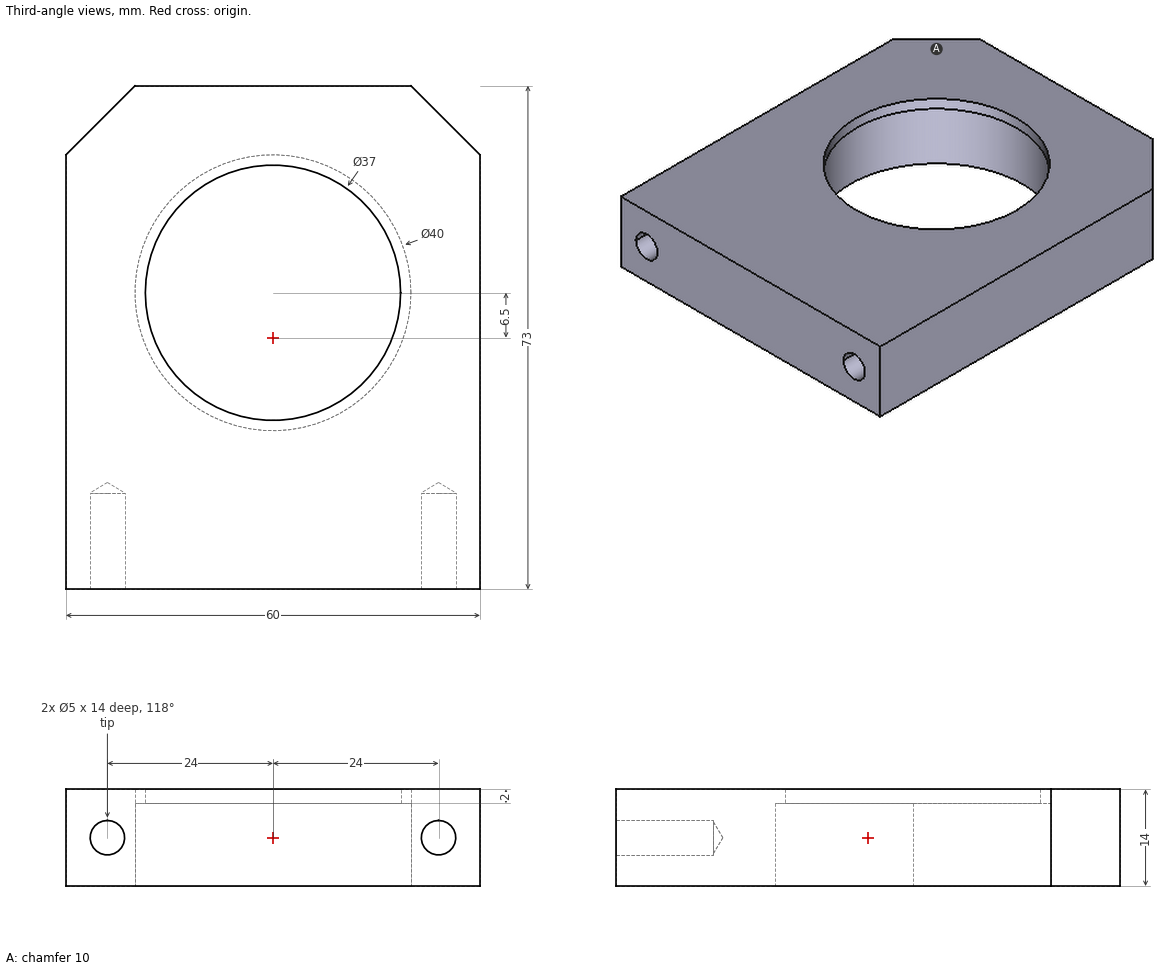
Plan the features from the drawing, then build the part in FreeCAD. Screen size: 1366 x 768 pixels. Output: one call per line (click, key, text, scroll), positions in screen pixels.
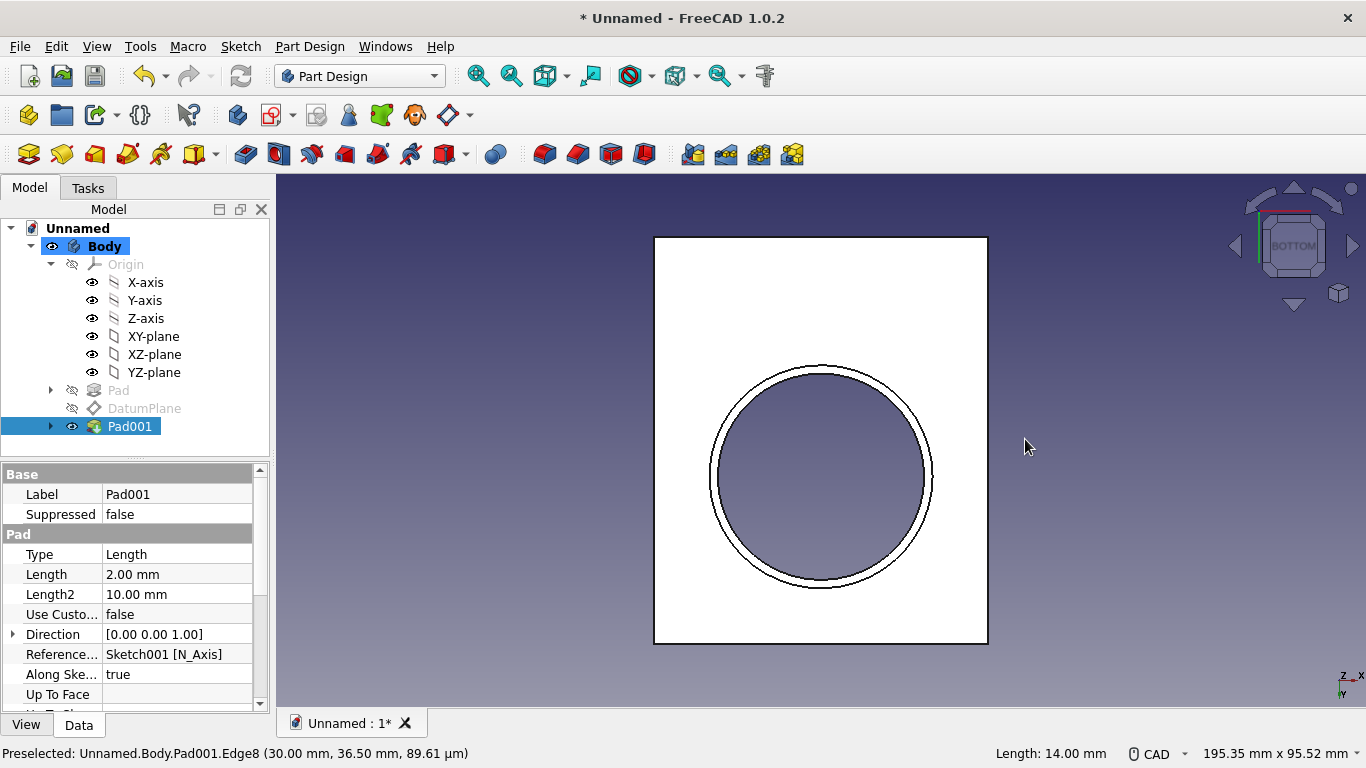
key(4)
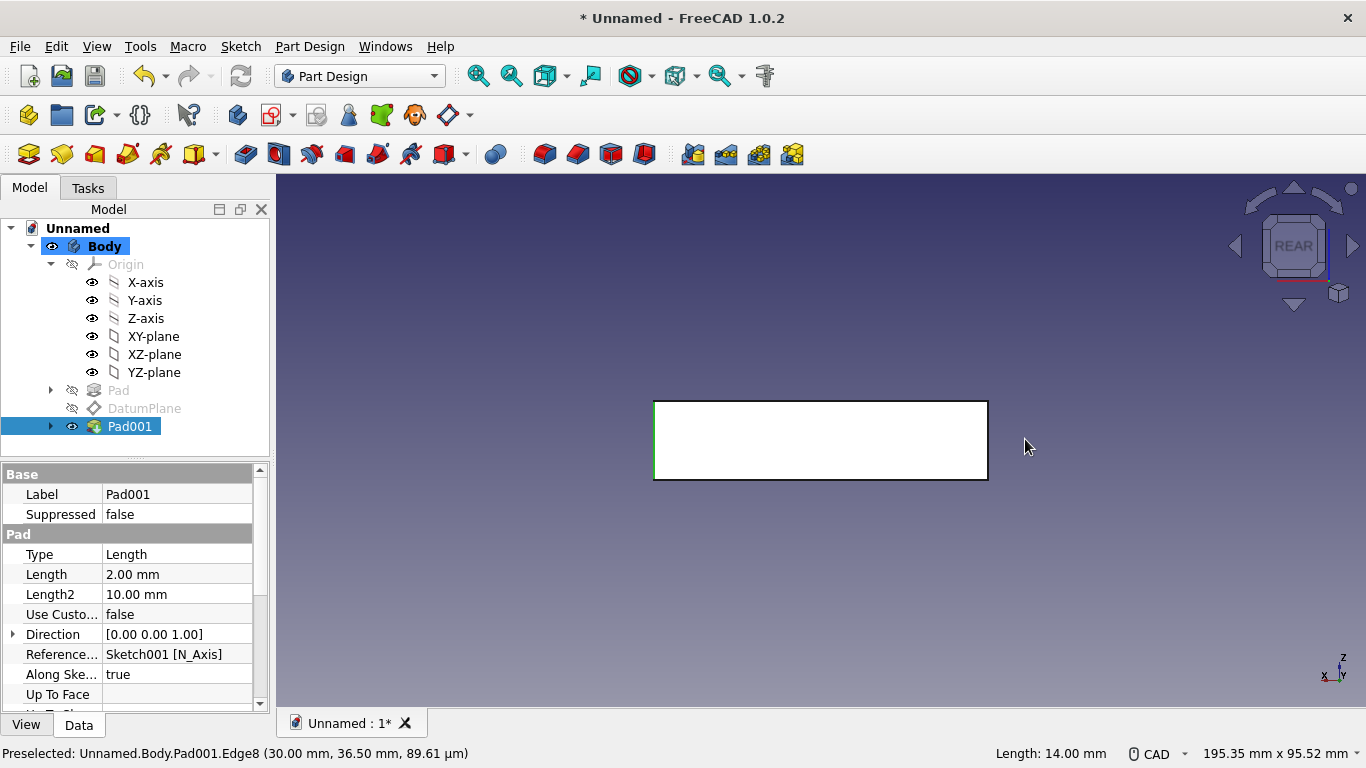
click(479, 76)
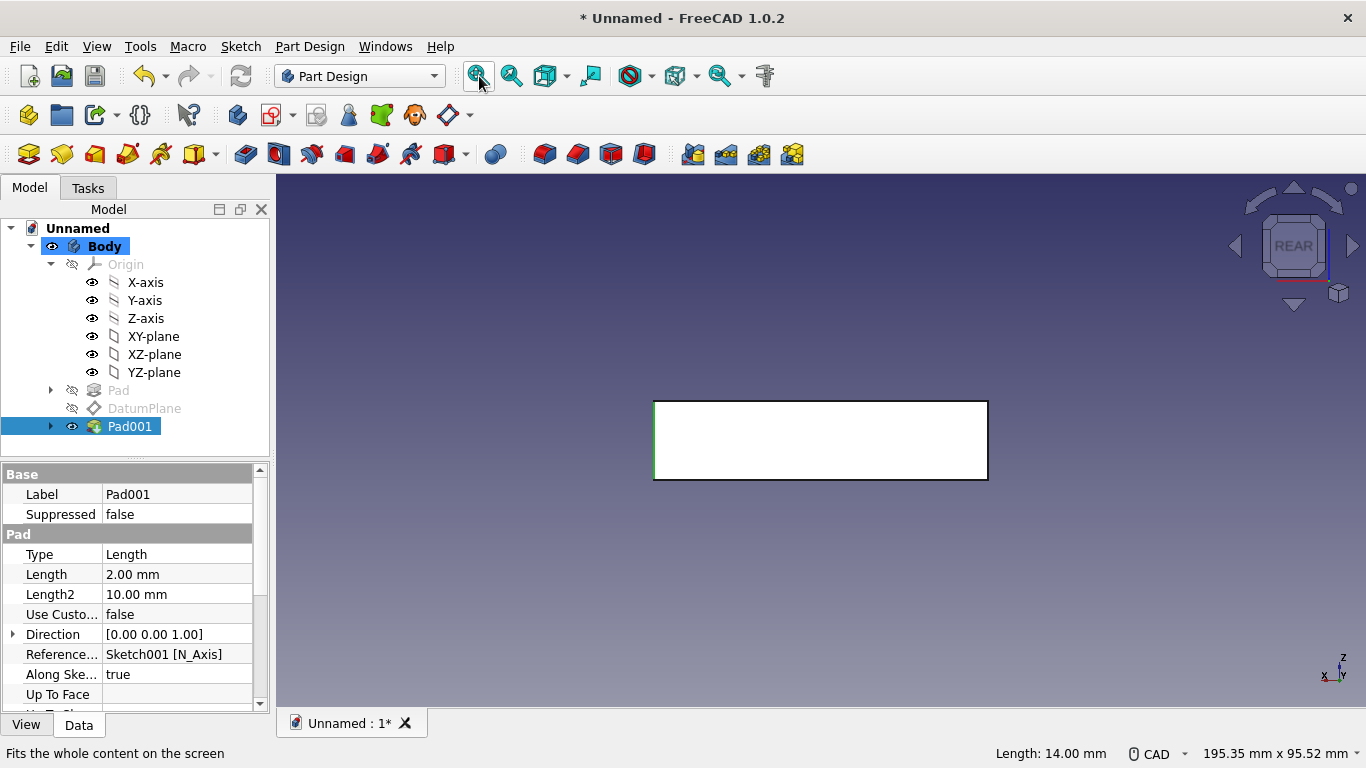
click(988, 440, ctrl)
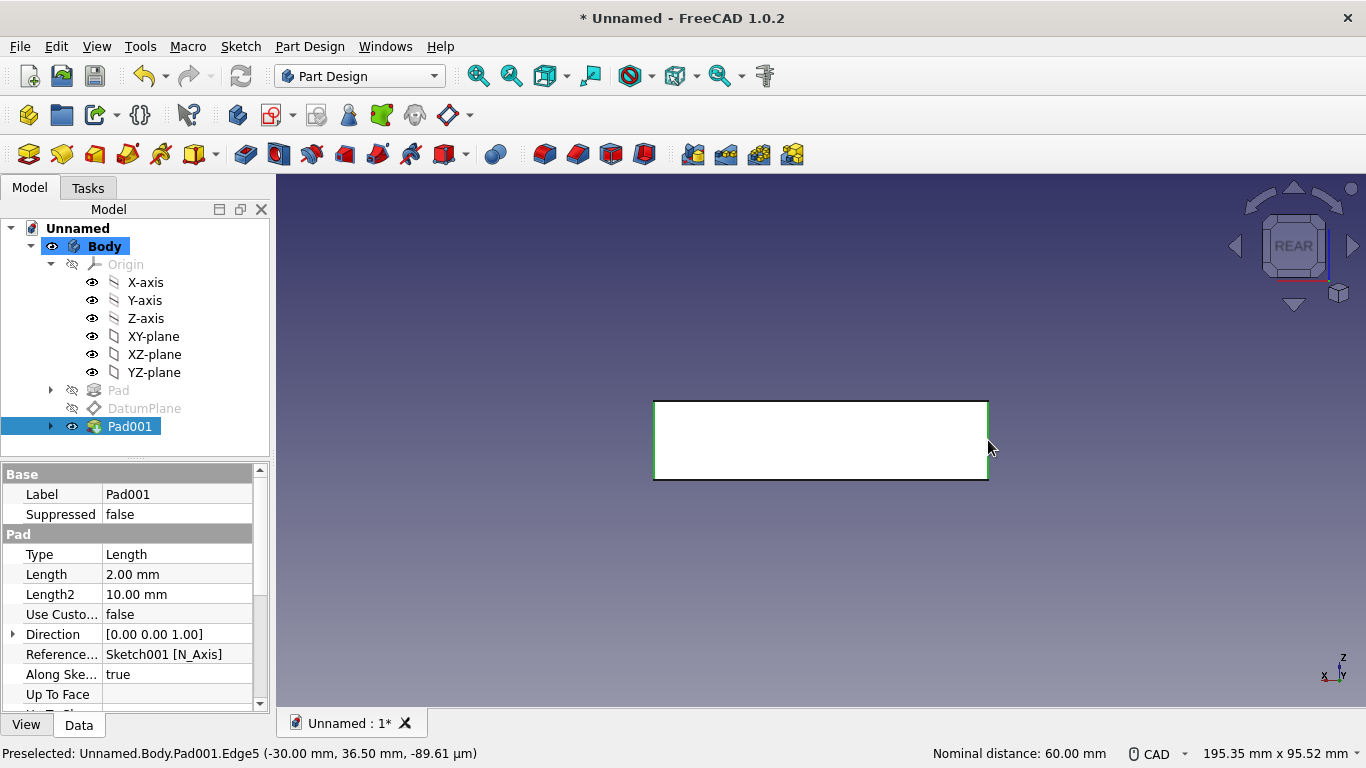
click(578, 154)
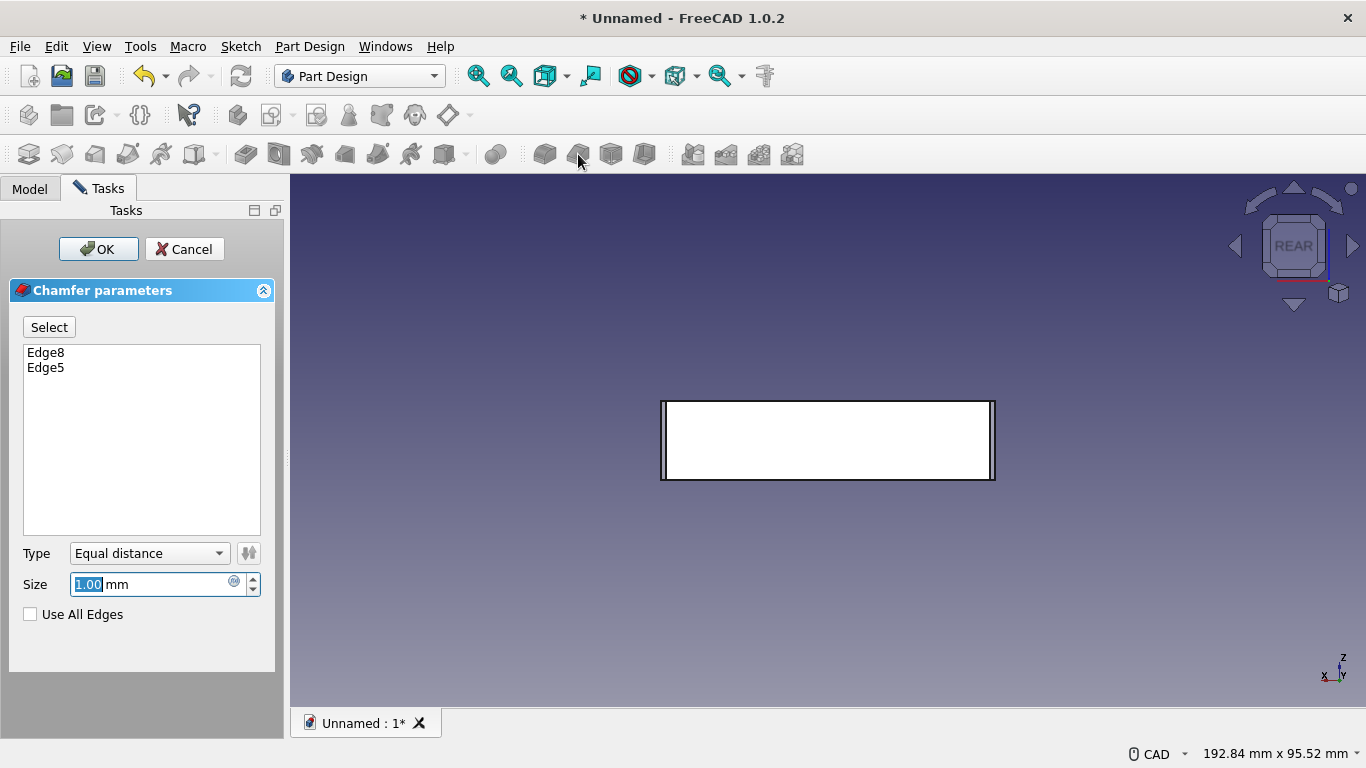
text(10)
key(Tab)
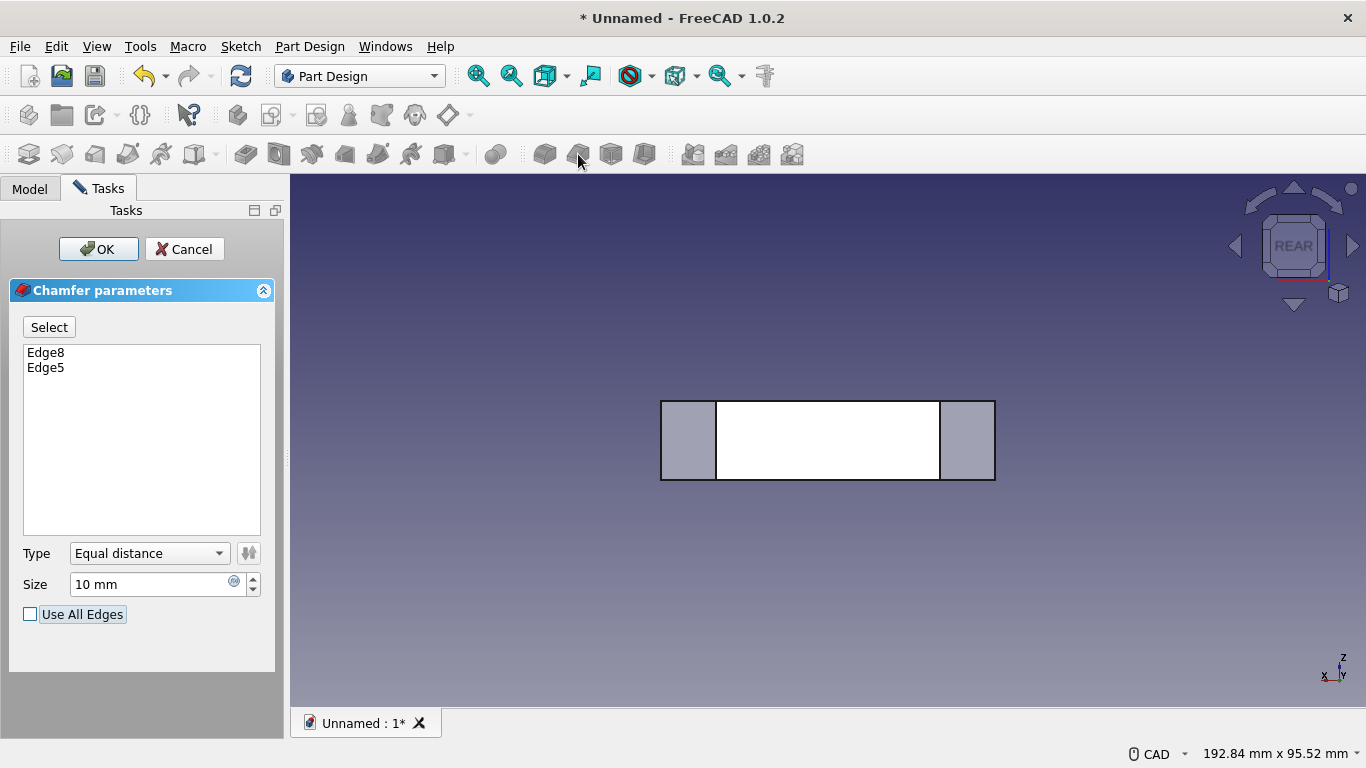
click(99, 249)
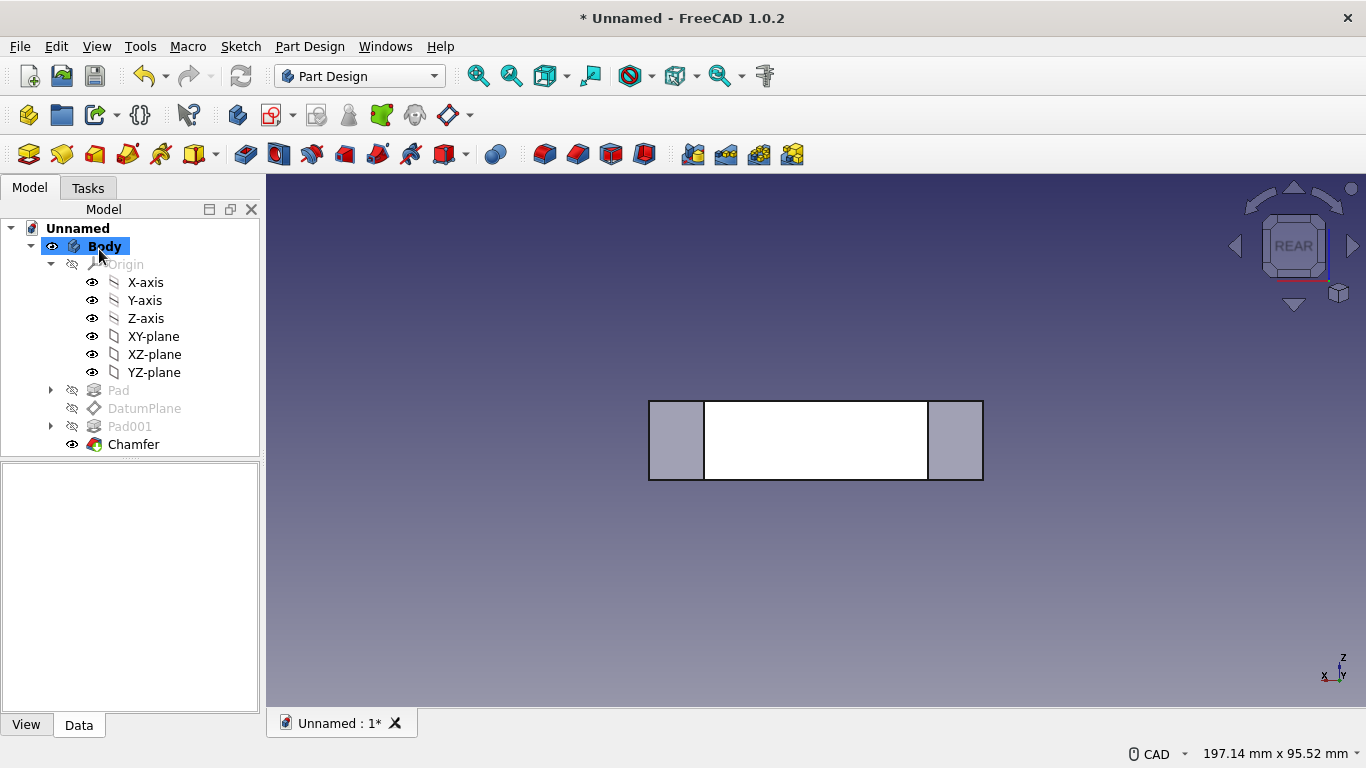
click(479, 76)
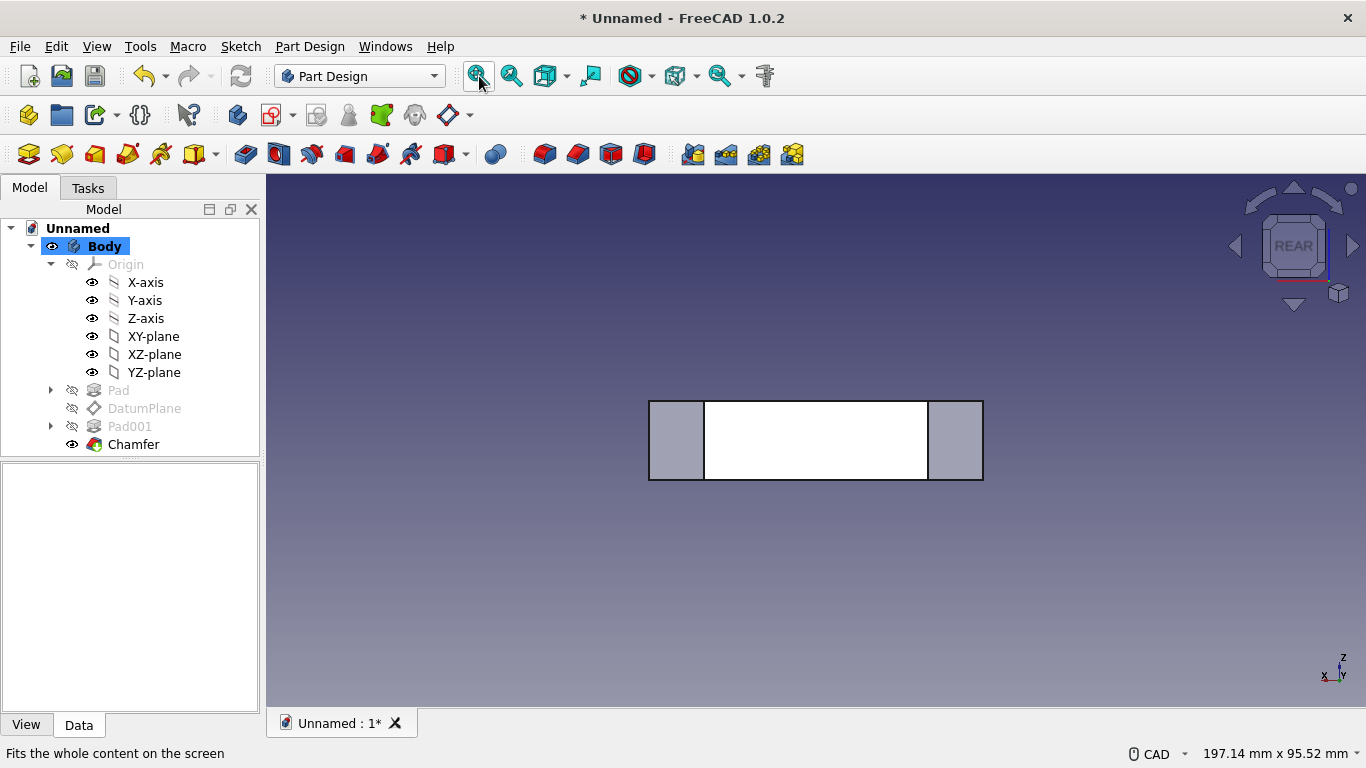
key(0)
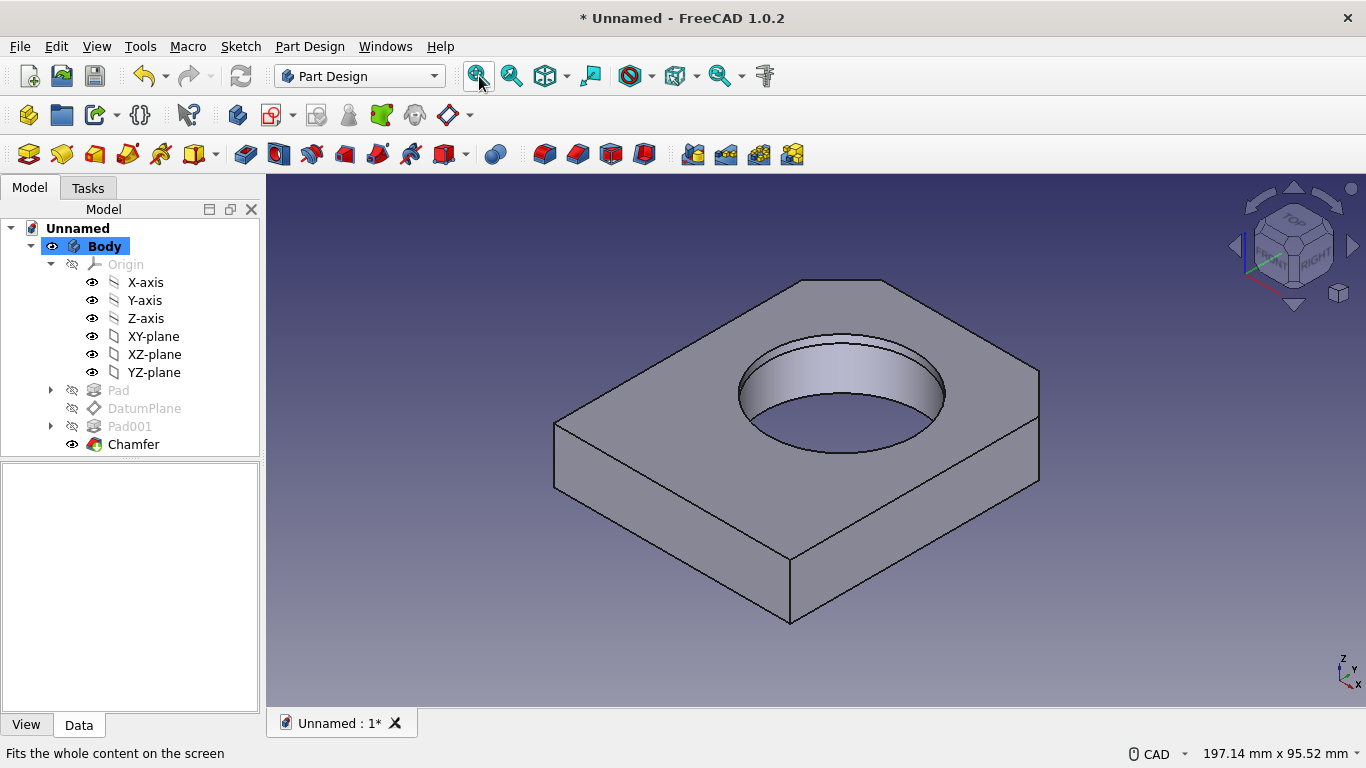
click(740, 562)